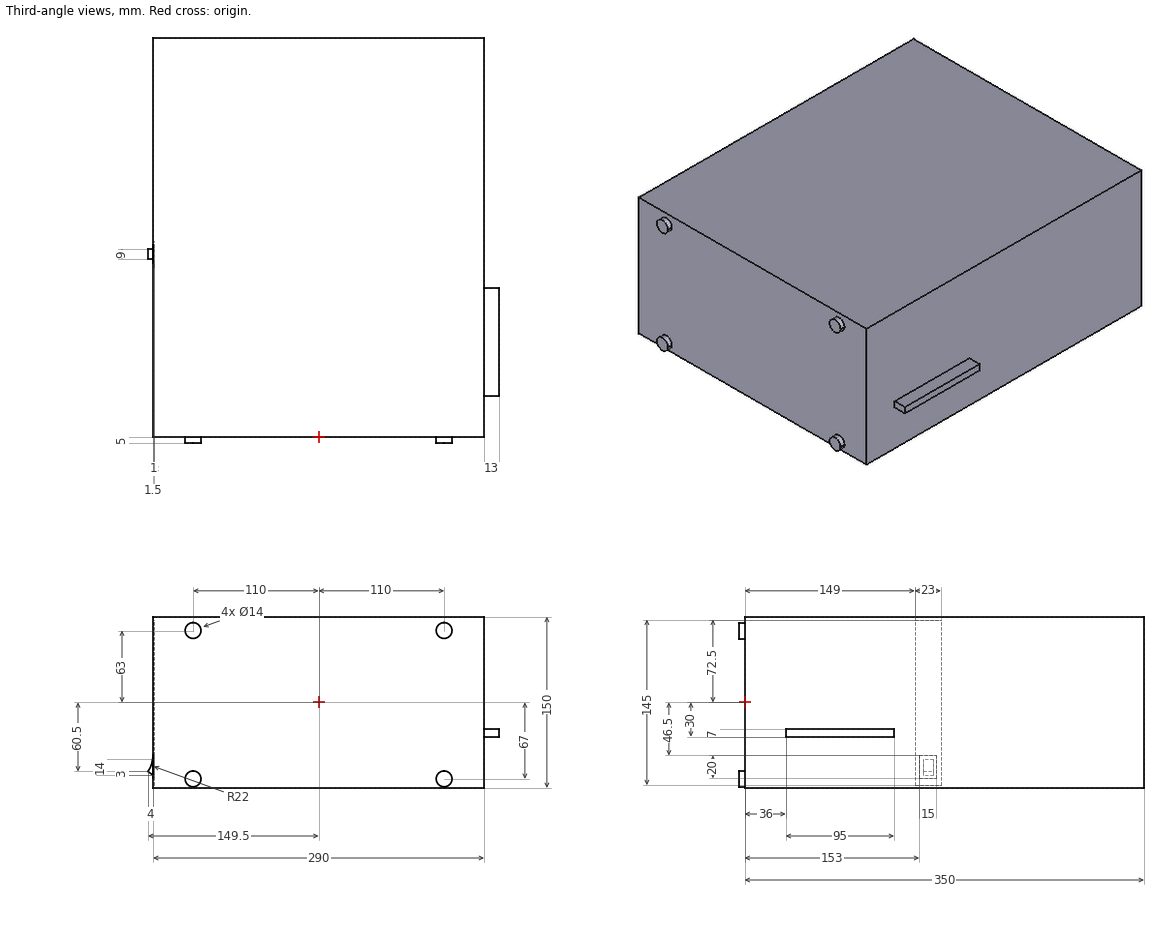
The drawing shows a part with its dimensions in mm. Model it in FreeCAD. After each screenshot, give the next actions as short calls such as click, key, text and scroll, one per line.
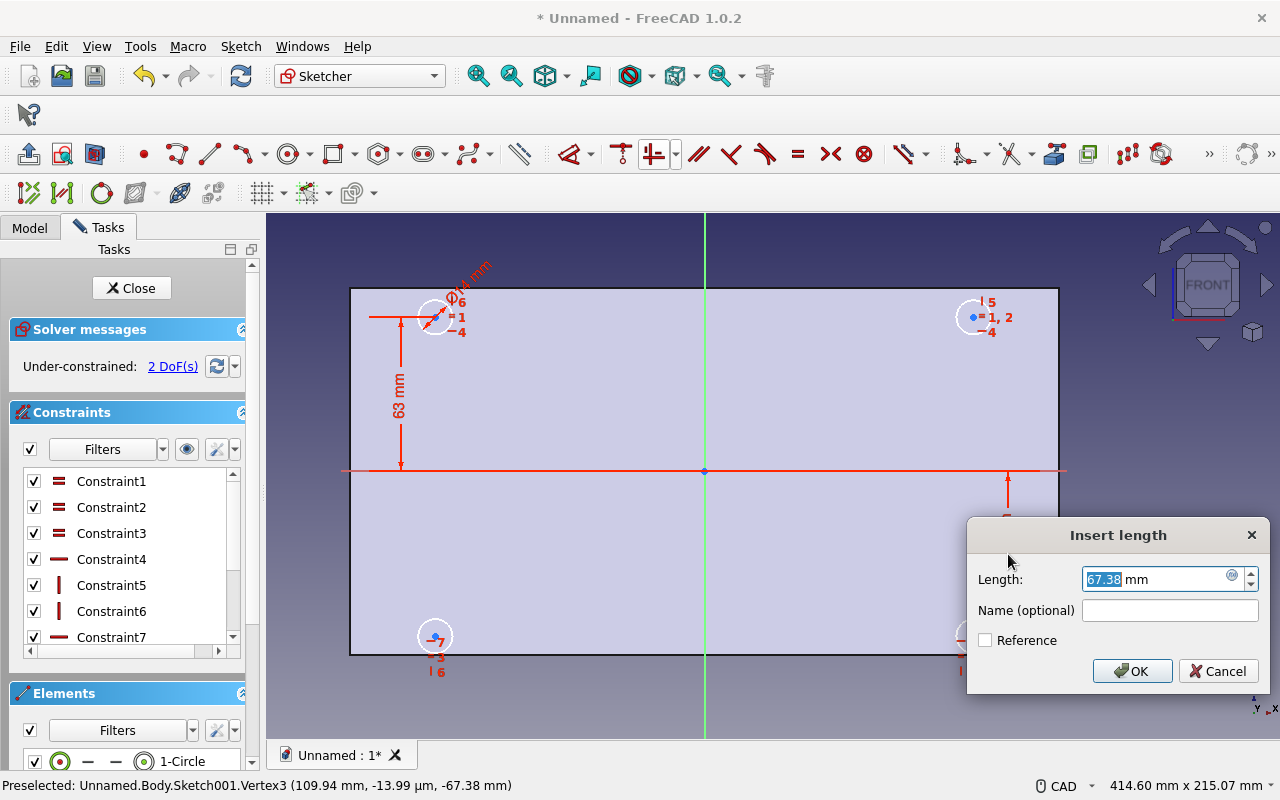
text(67)
key(Return)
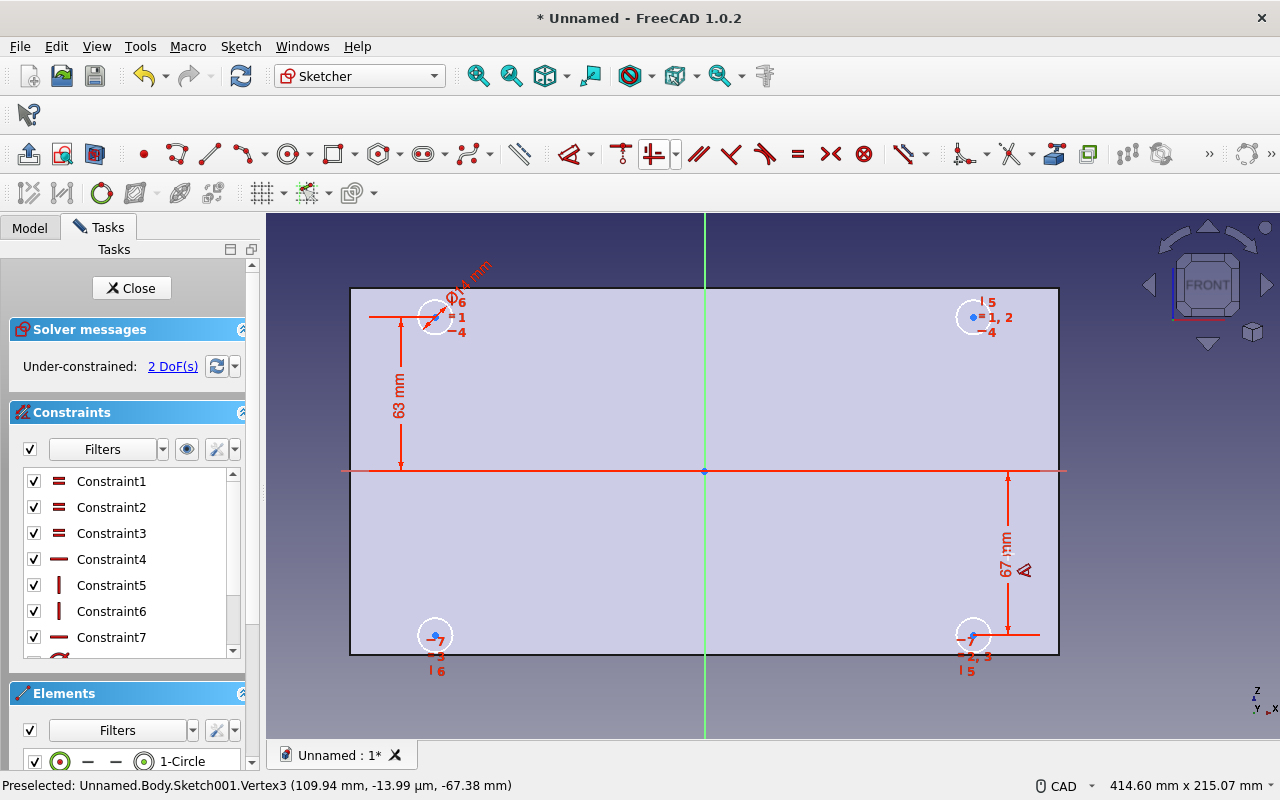
click(435, 317)
click(570, 283)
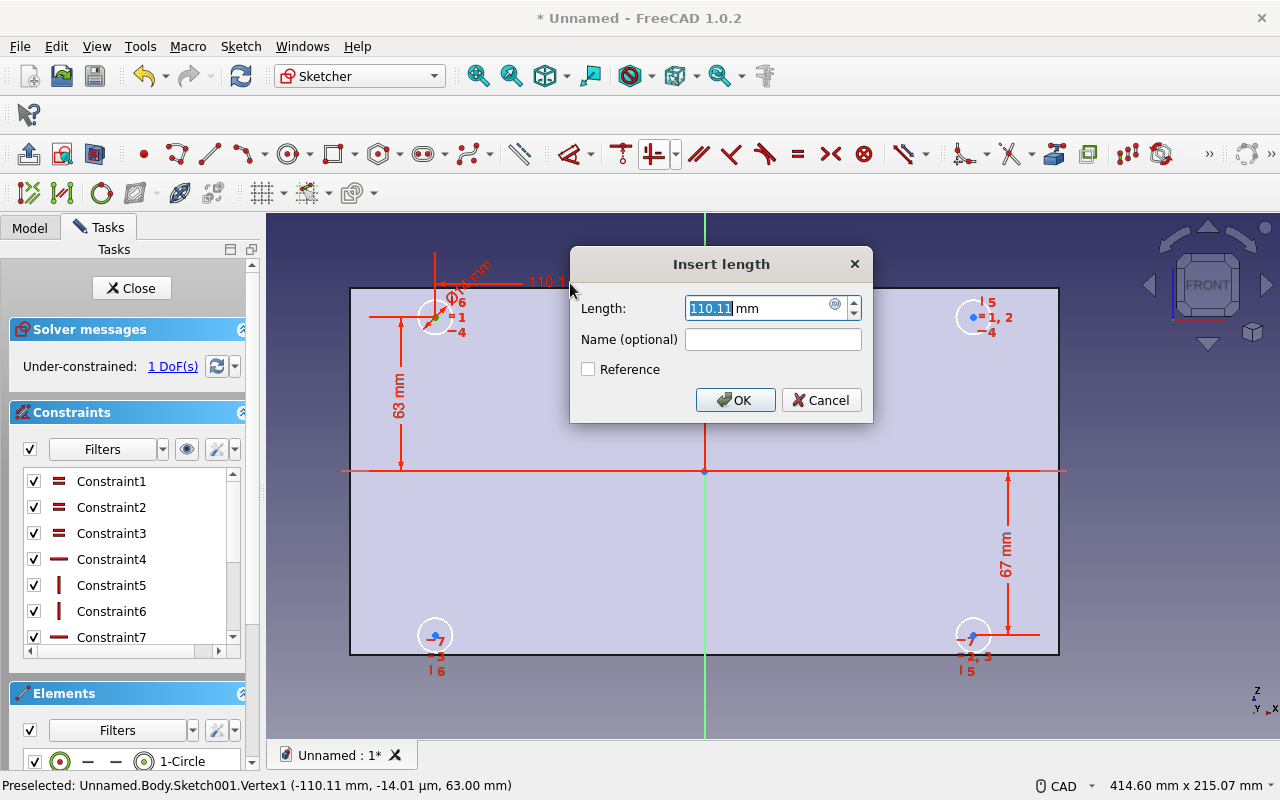
text(110)
key(Return)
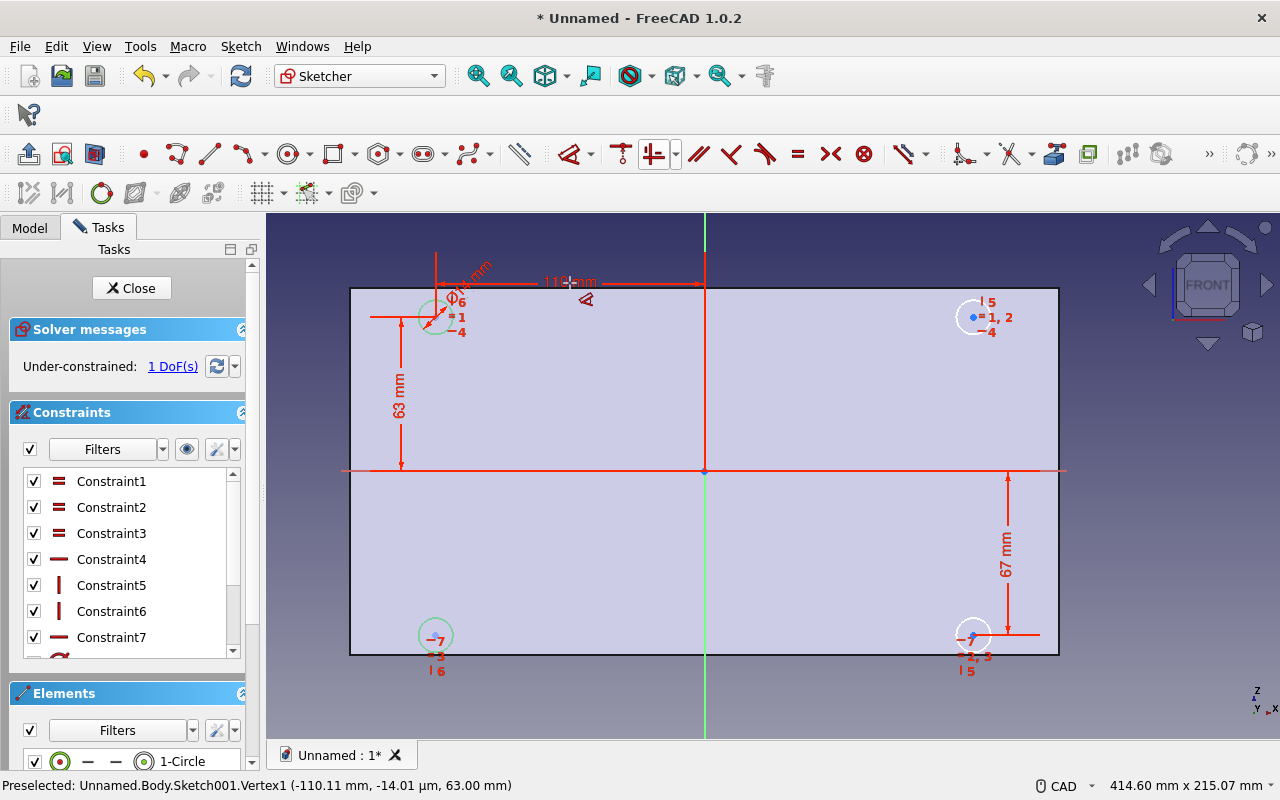
click(974, 317)
click(839, 283)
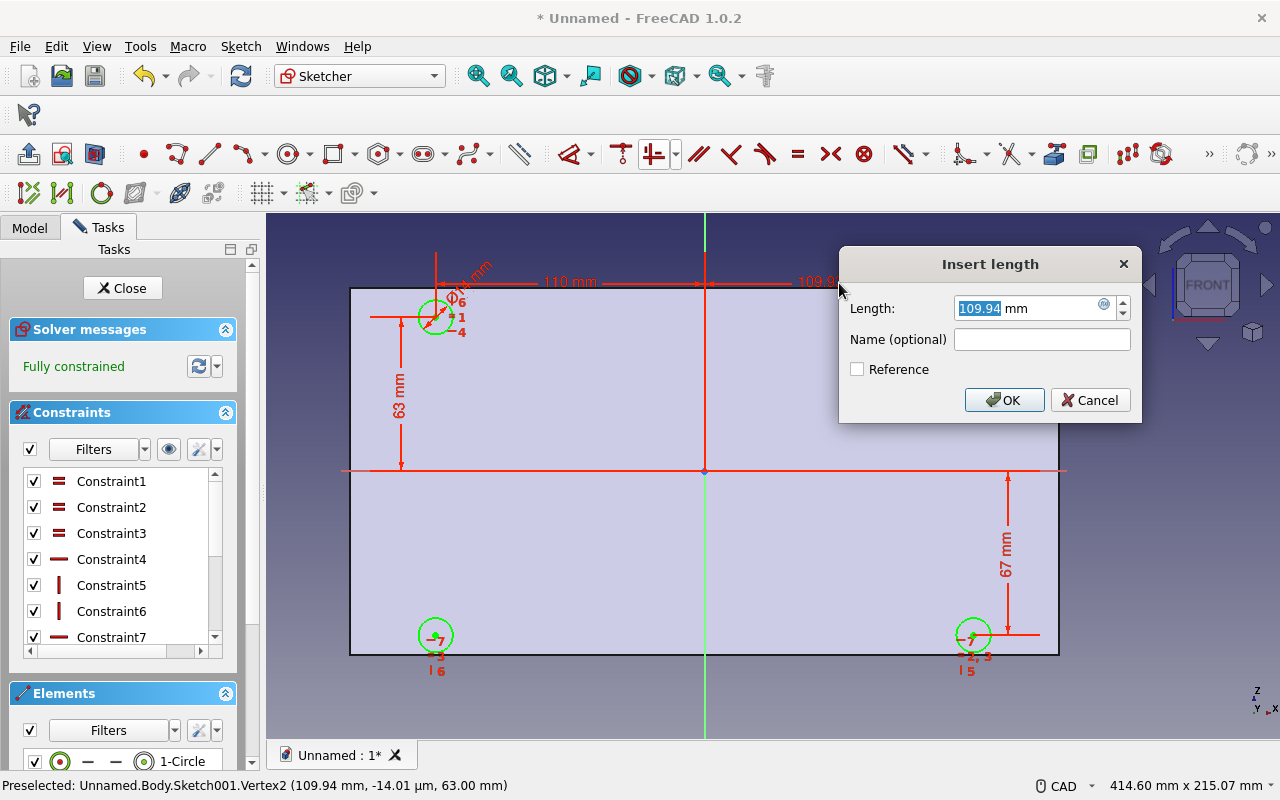
text(110)
key(Return)
key(Escape)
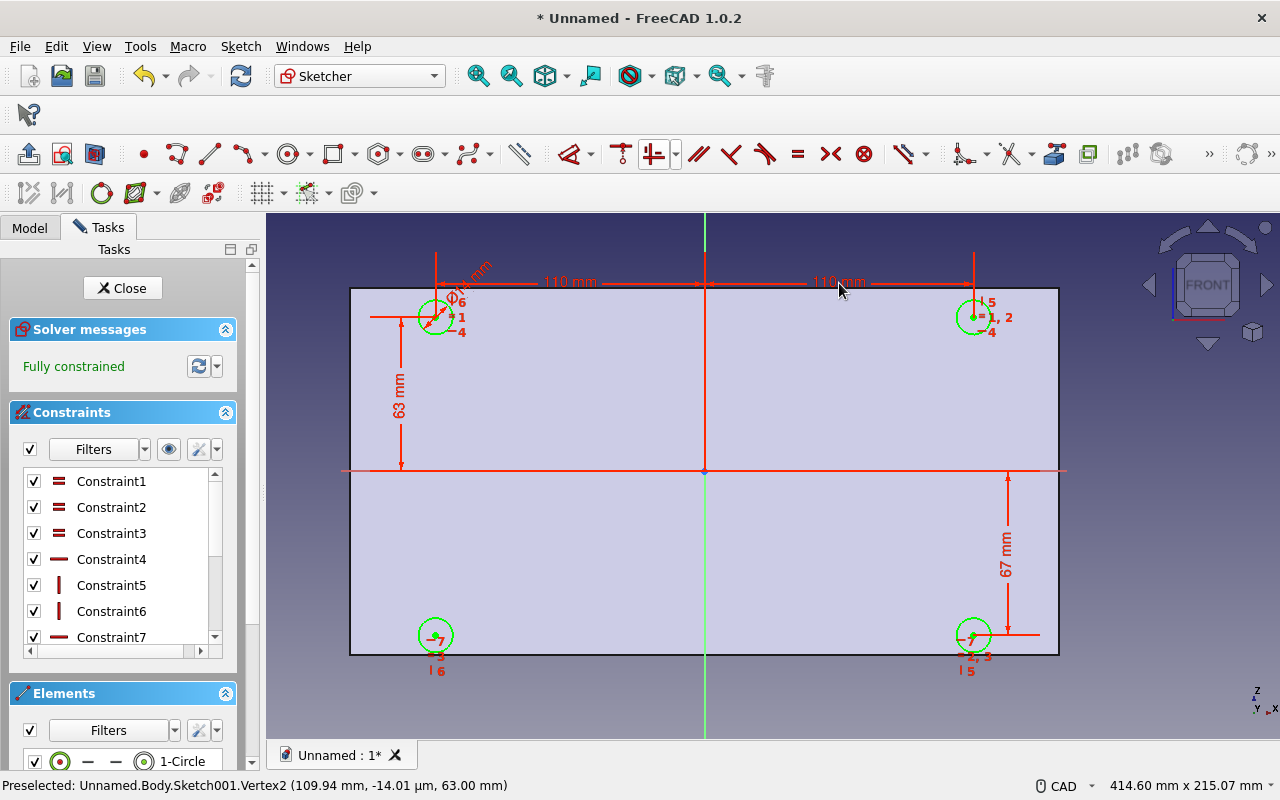
click(123, 288)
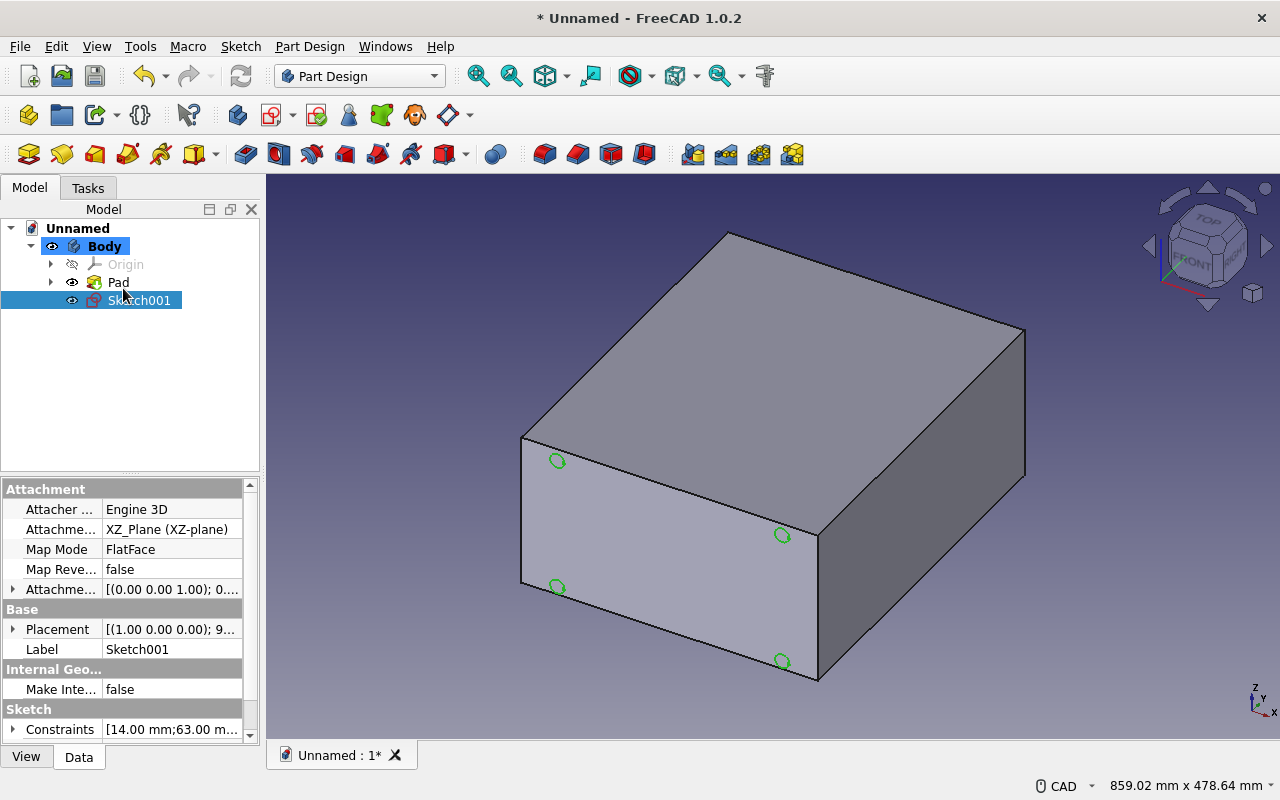
click(29, 154)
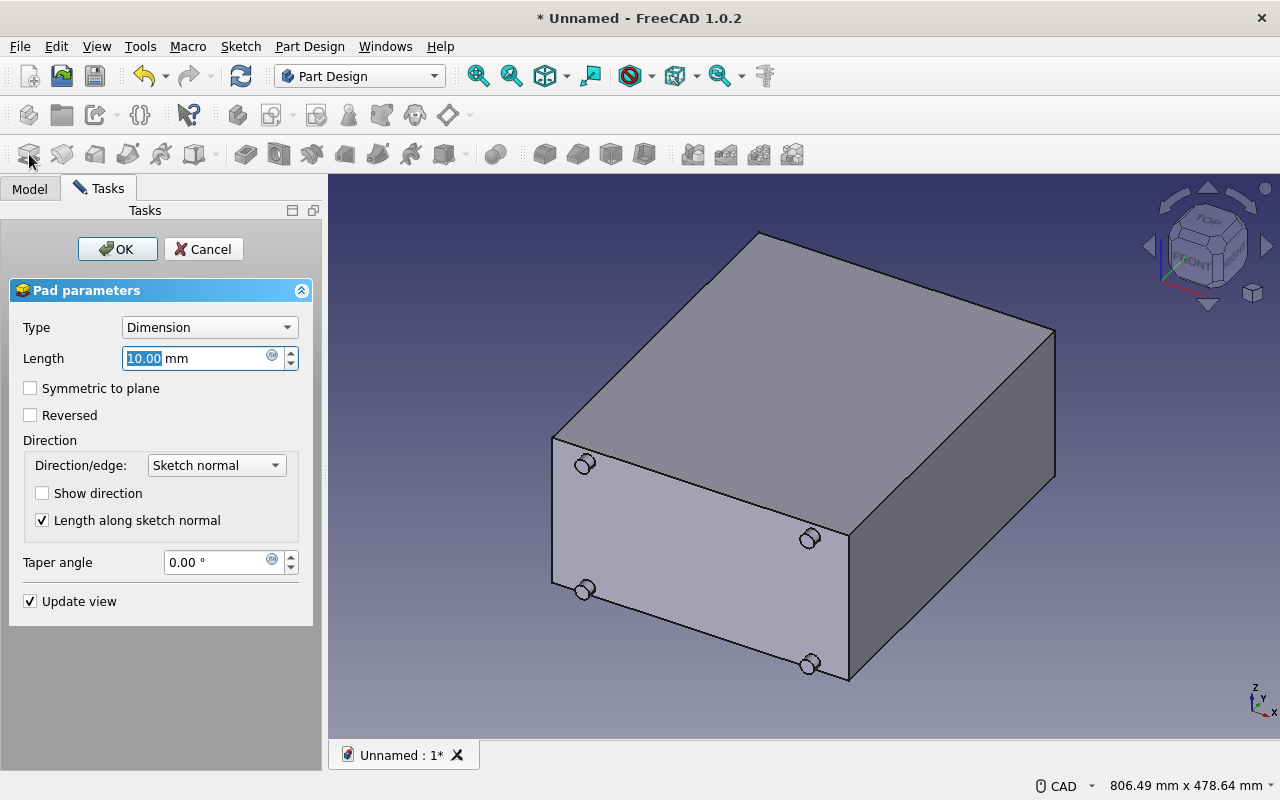
text(5)
key(Tab)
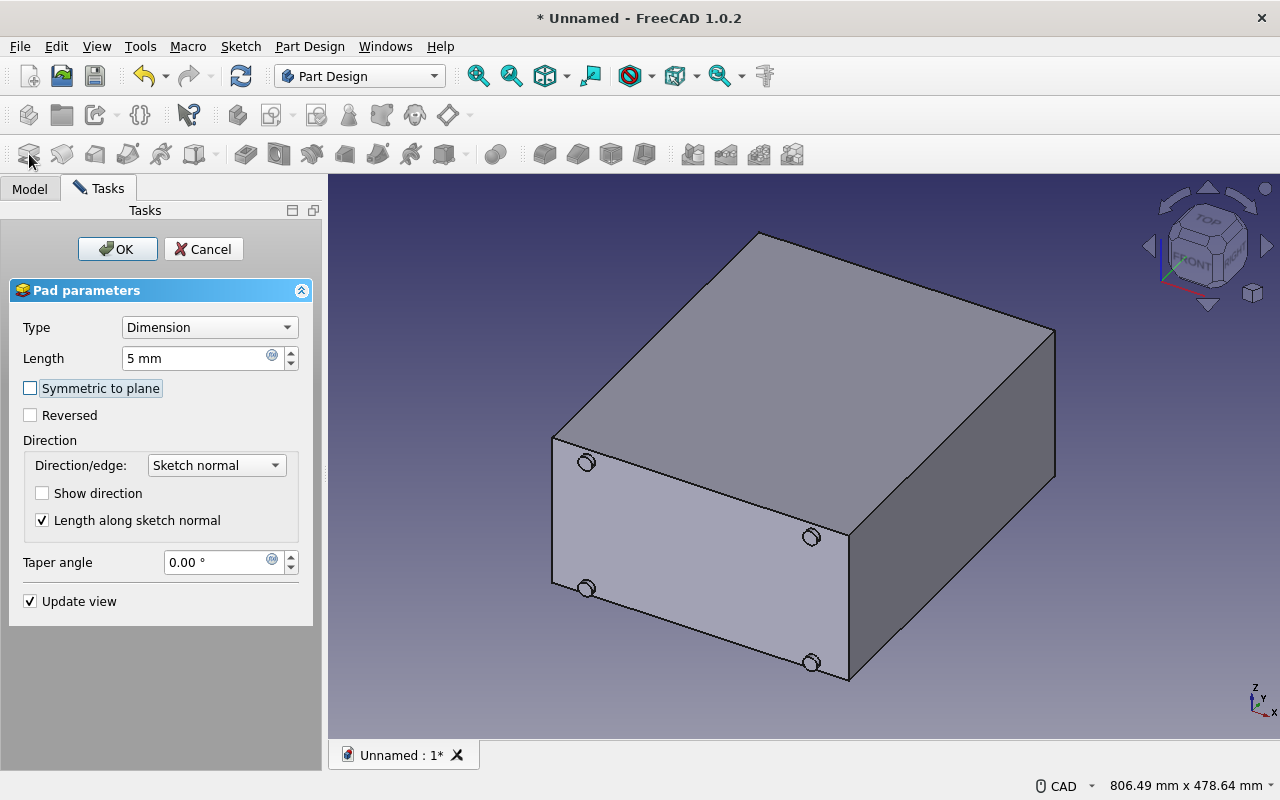
click(118, 249)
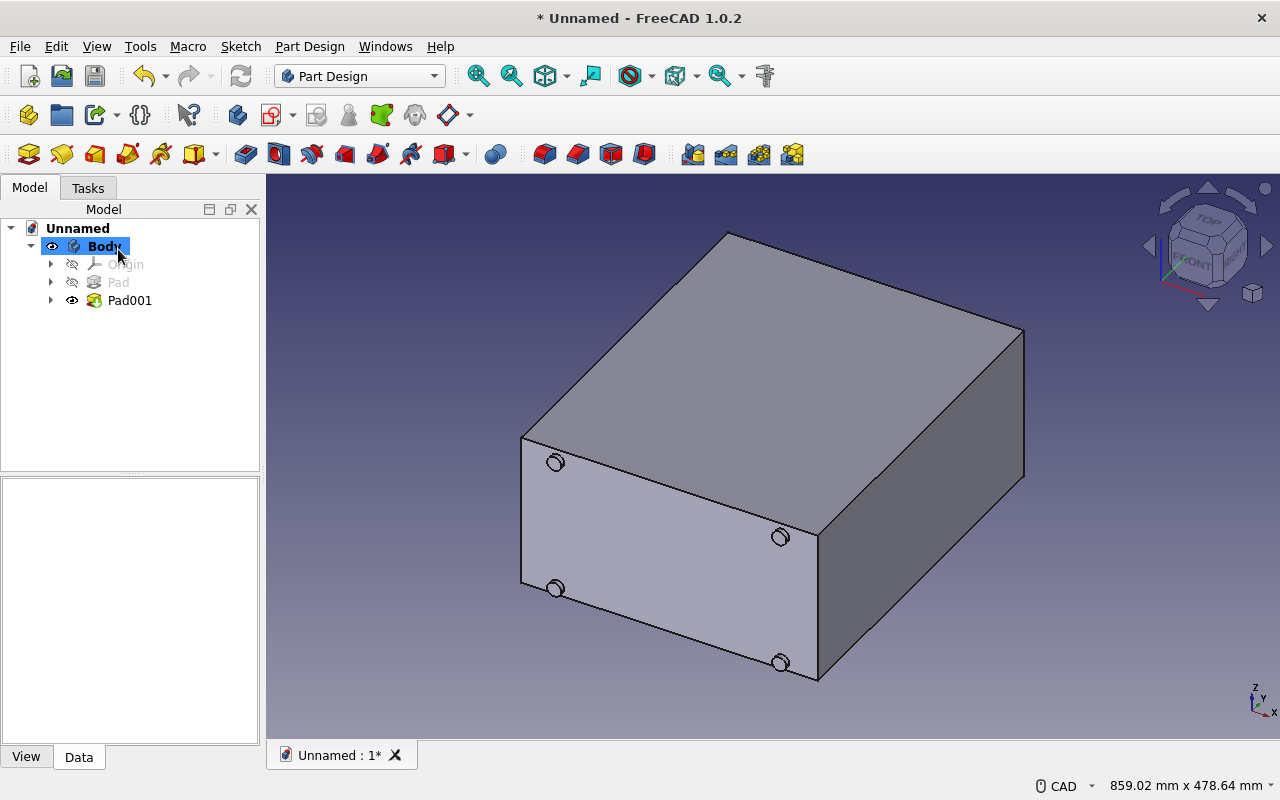
key(6)